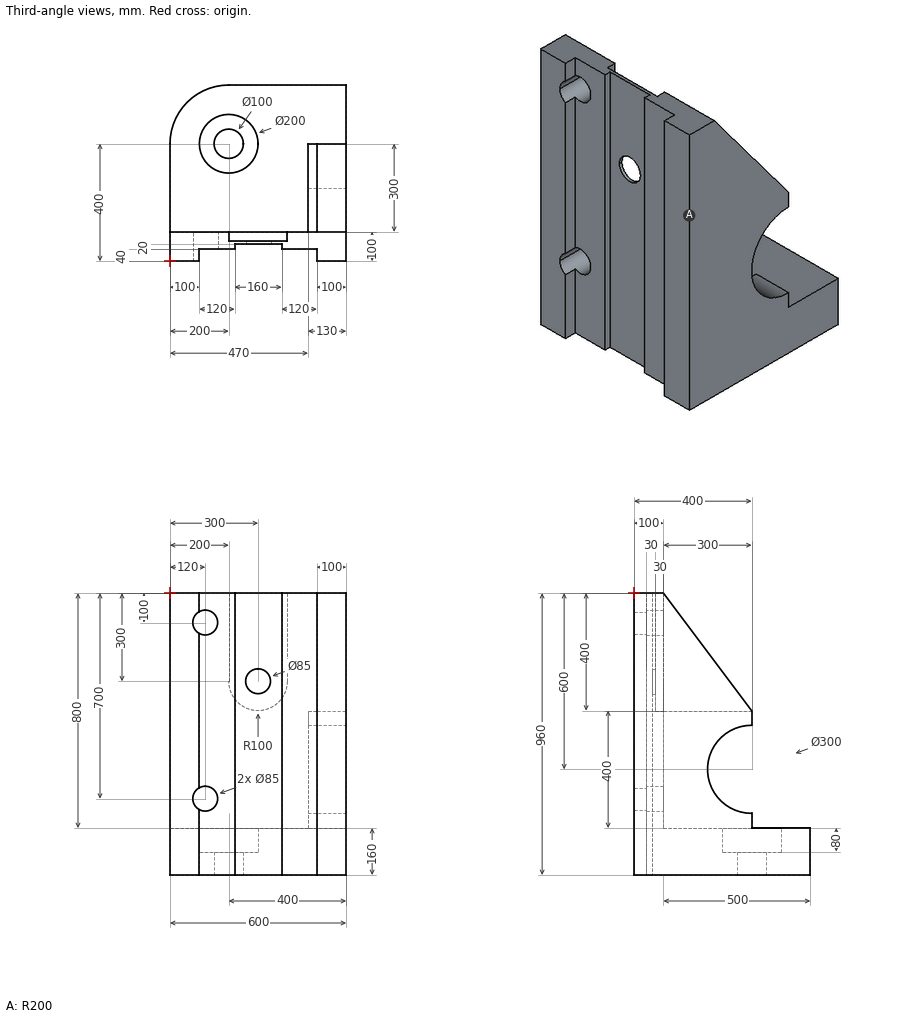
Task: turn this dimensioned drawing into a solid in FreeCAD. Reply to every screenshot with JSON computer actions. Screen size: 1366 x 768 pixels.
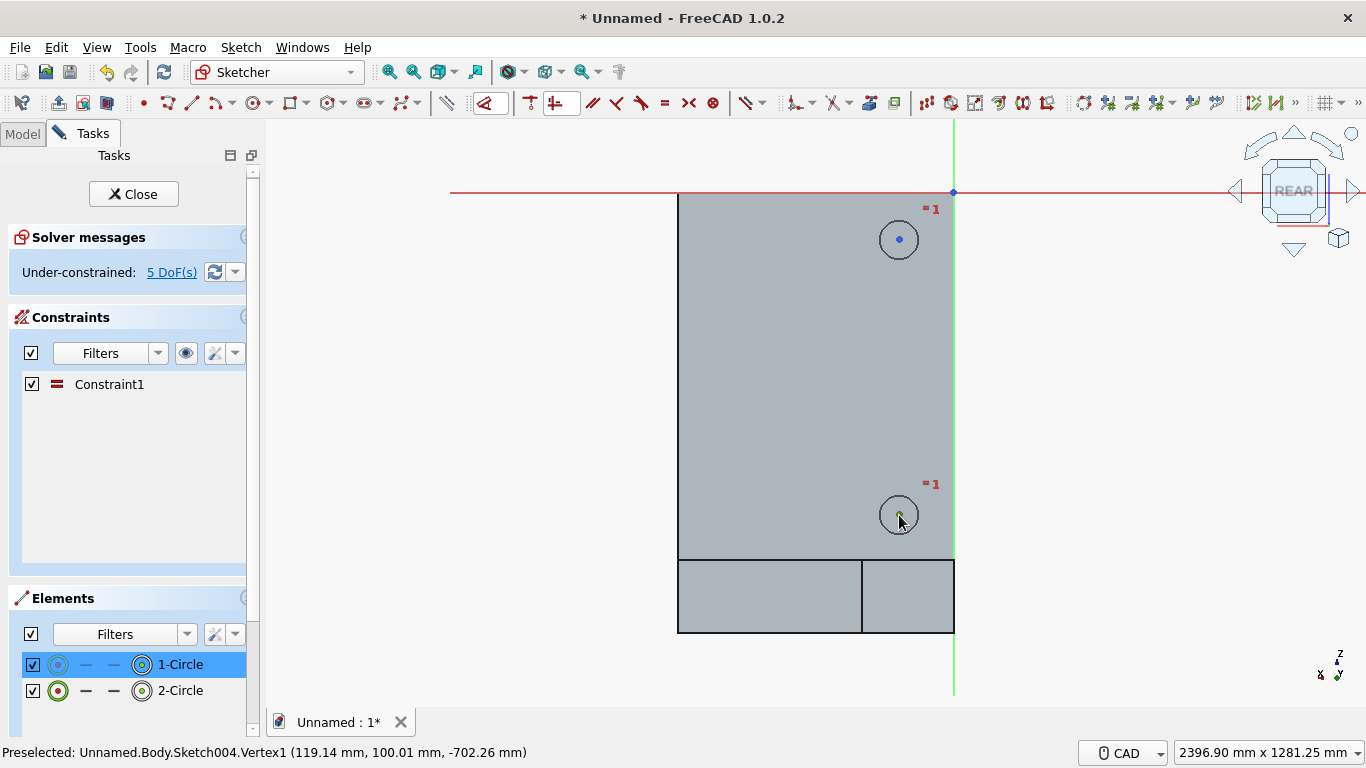
{"action": "left_click", "coordinate": [899, 240]}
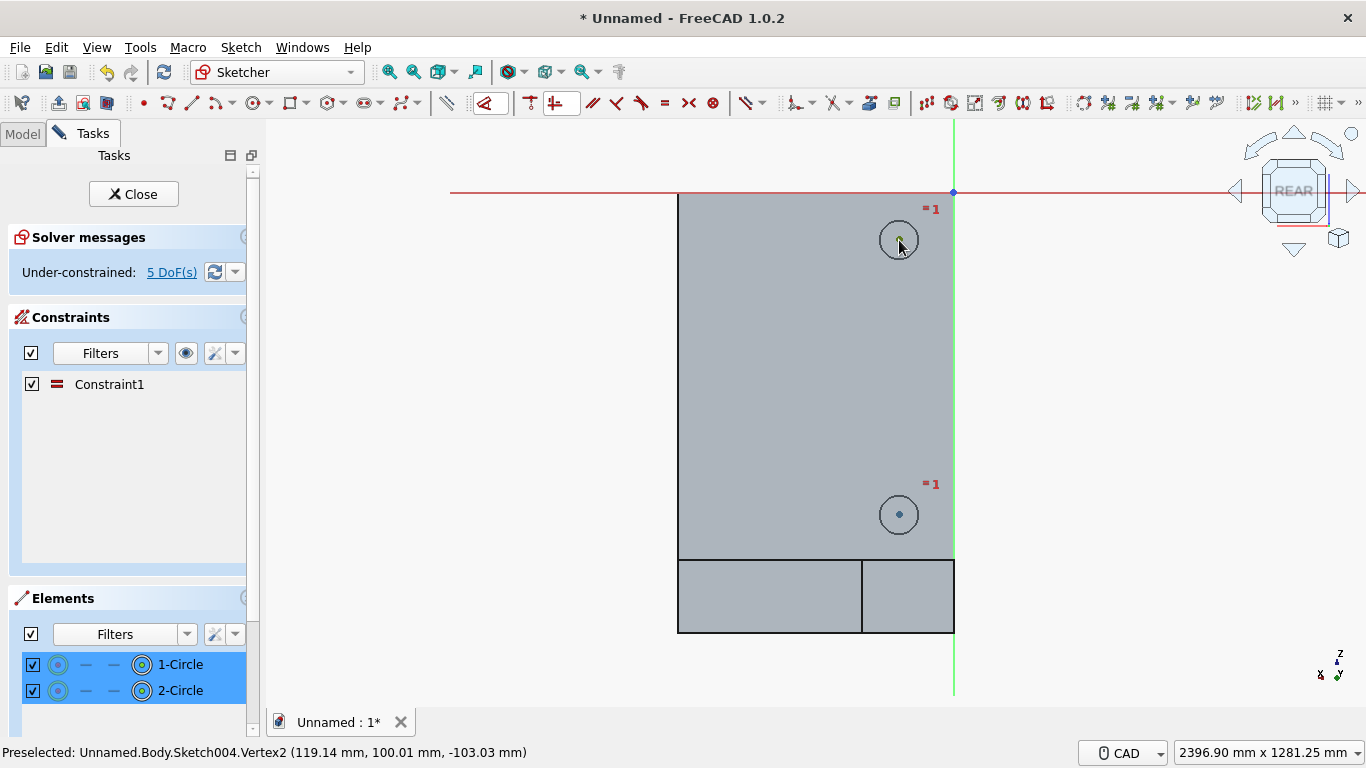
{"action": "key", "text": "v"}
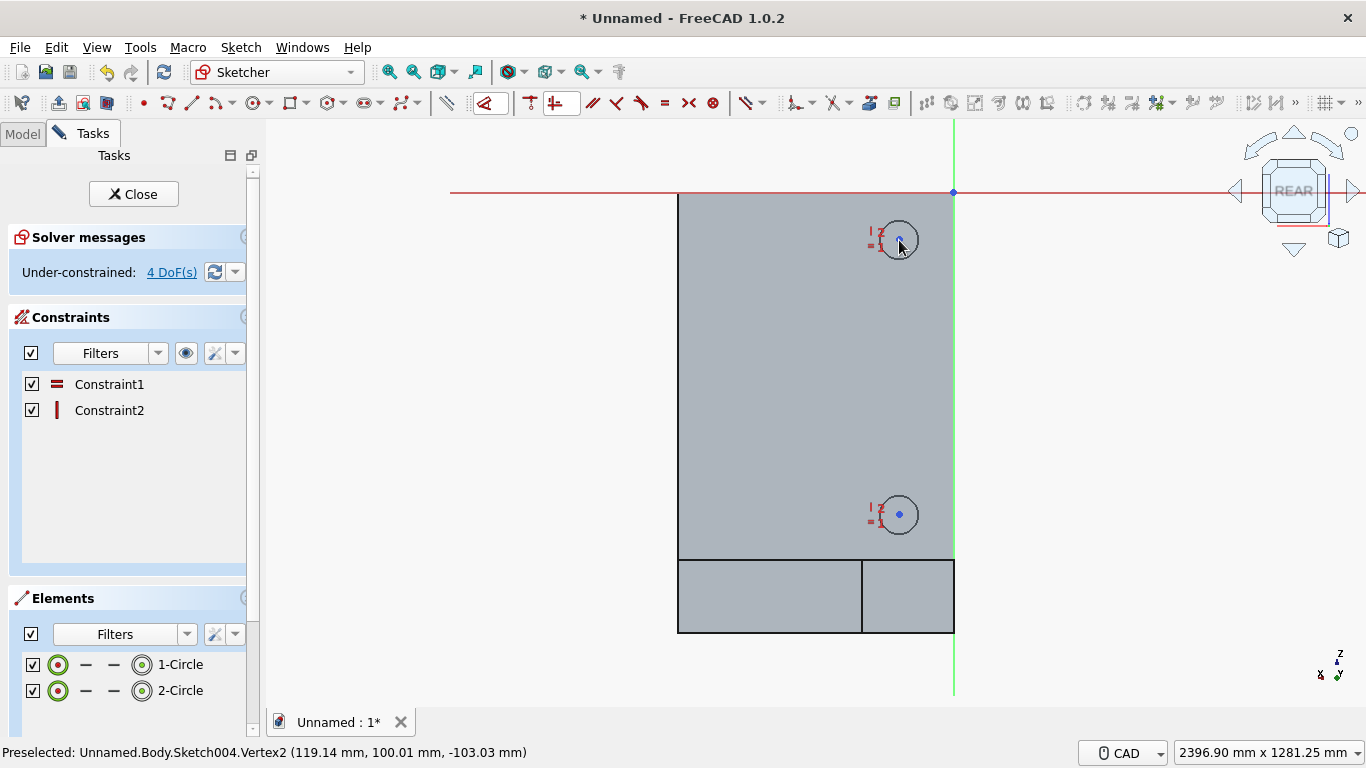
{"action": "left_click", "coordinate": [912, 501]}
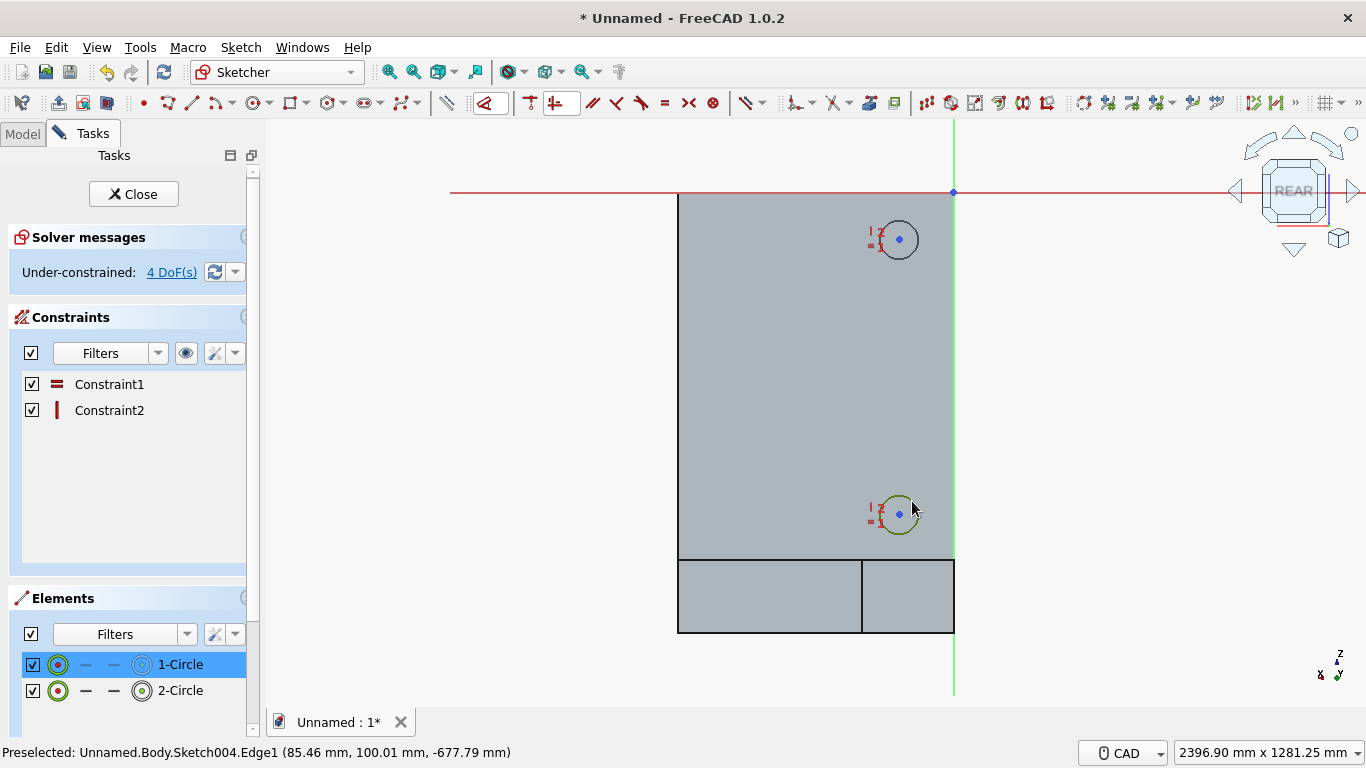
{"action": "key", "text": "k o"}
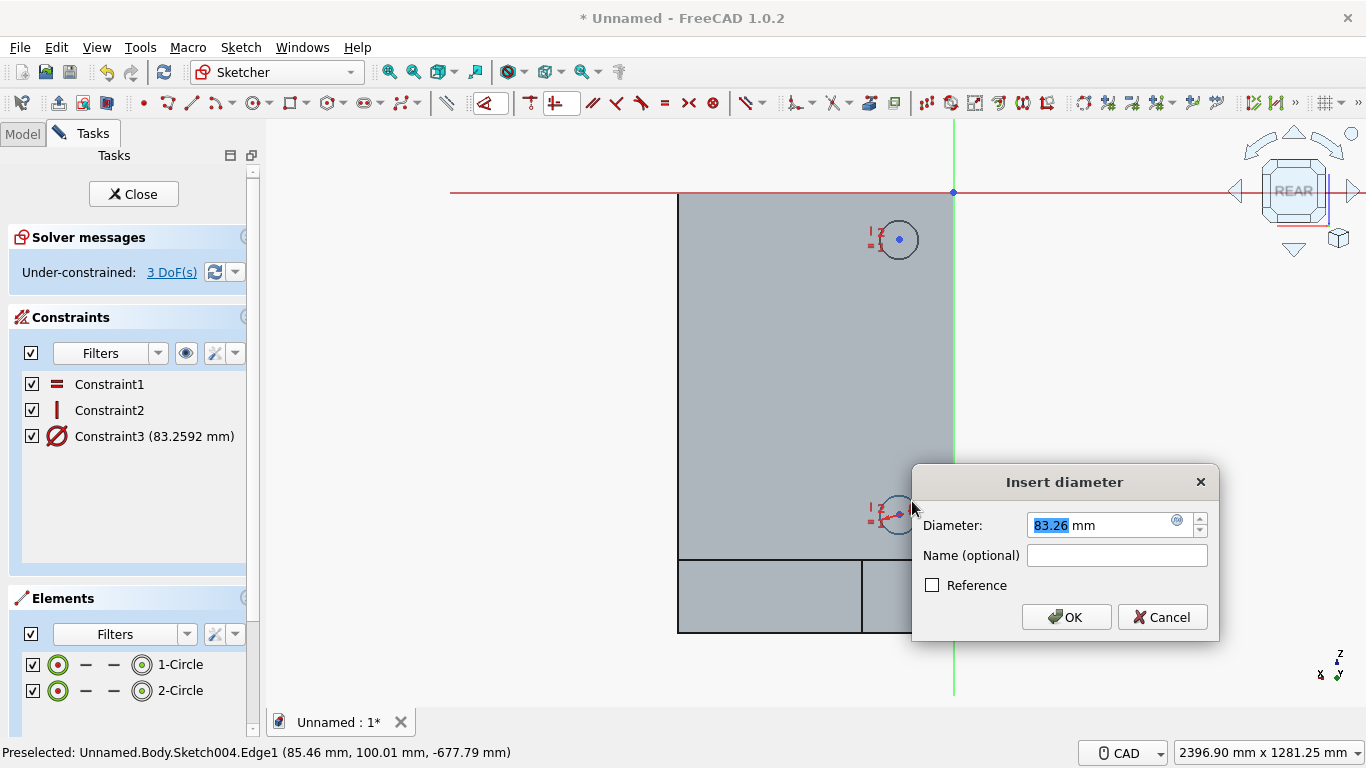
{"action": "type", "text": "85"}
{"action": "key", "text": "Return"}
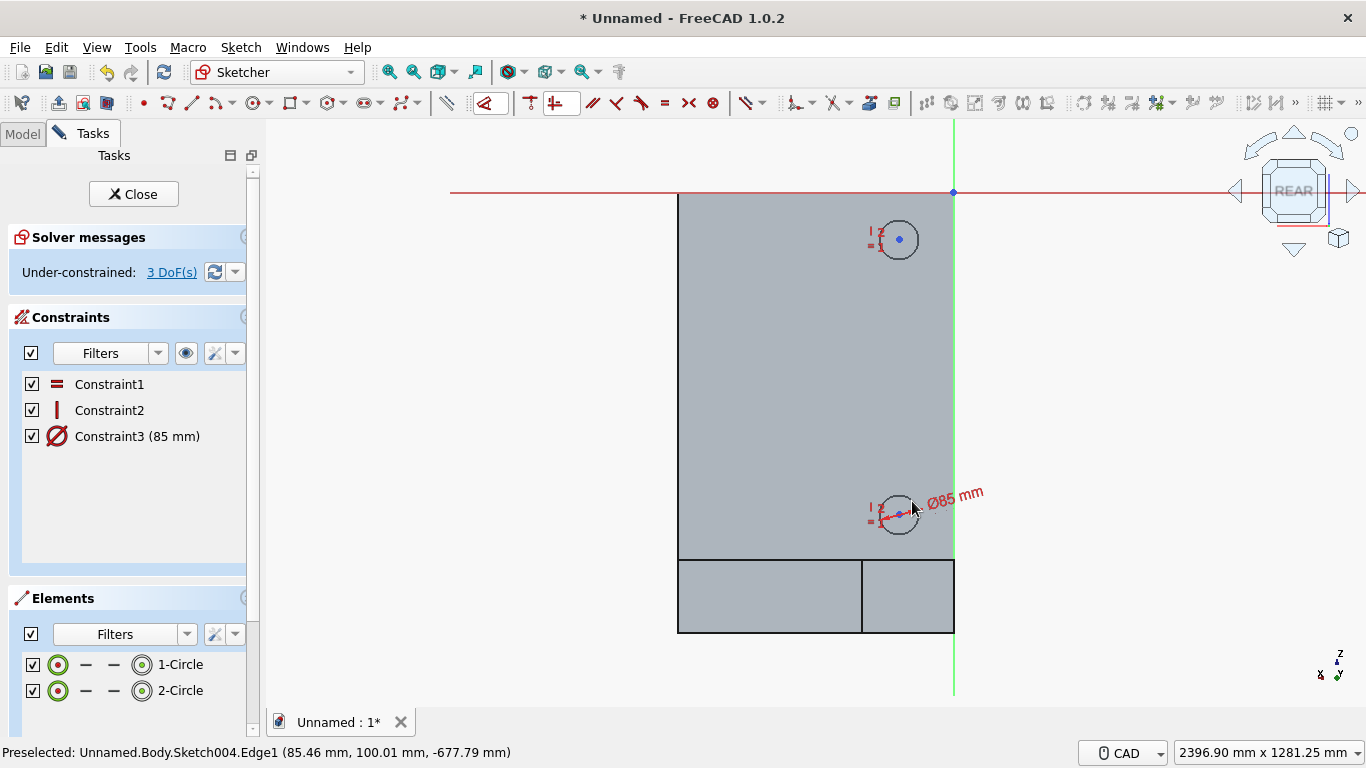
{"action": "left_click", "coordinate": [899, 515]}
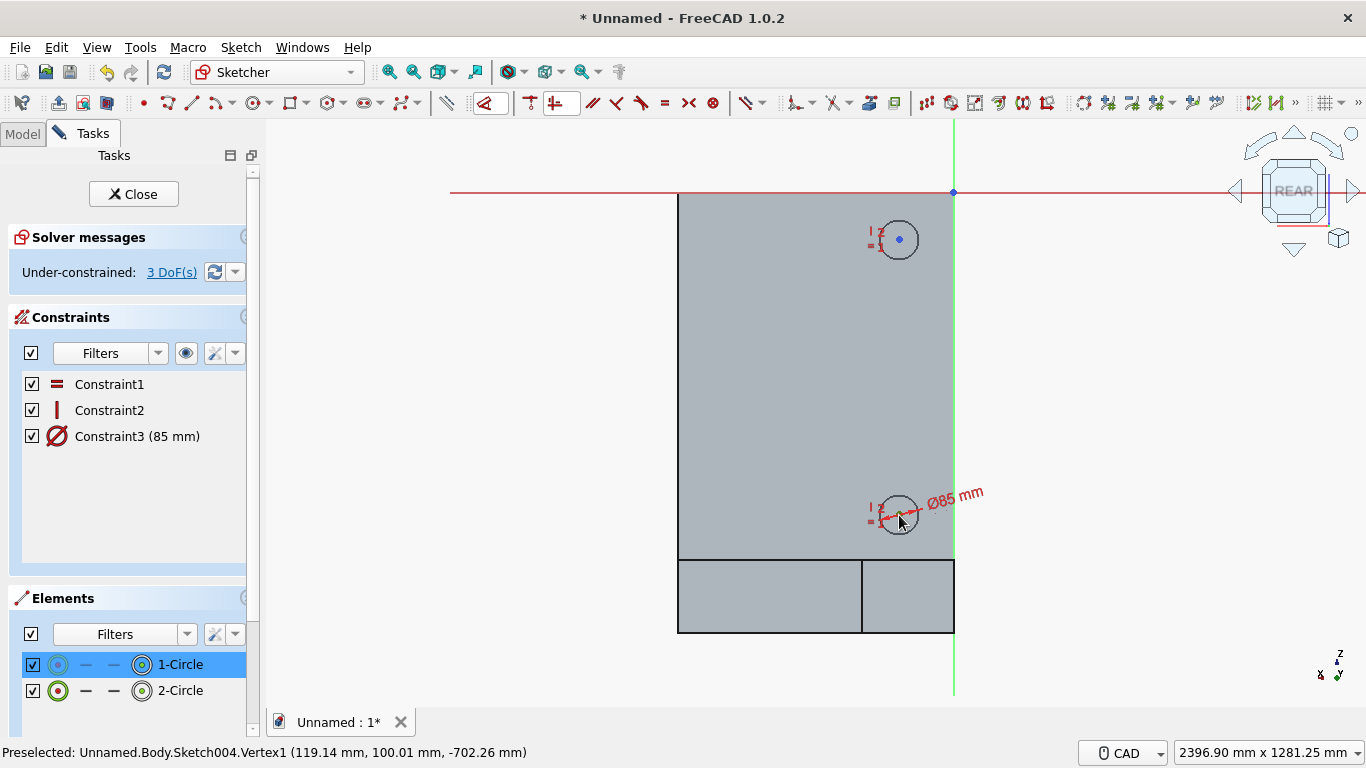
{"action": "left_click", "coordinate": [502, 104]}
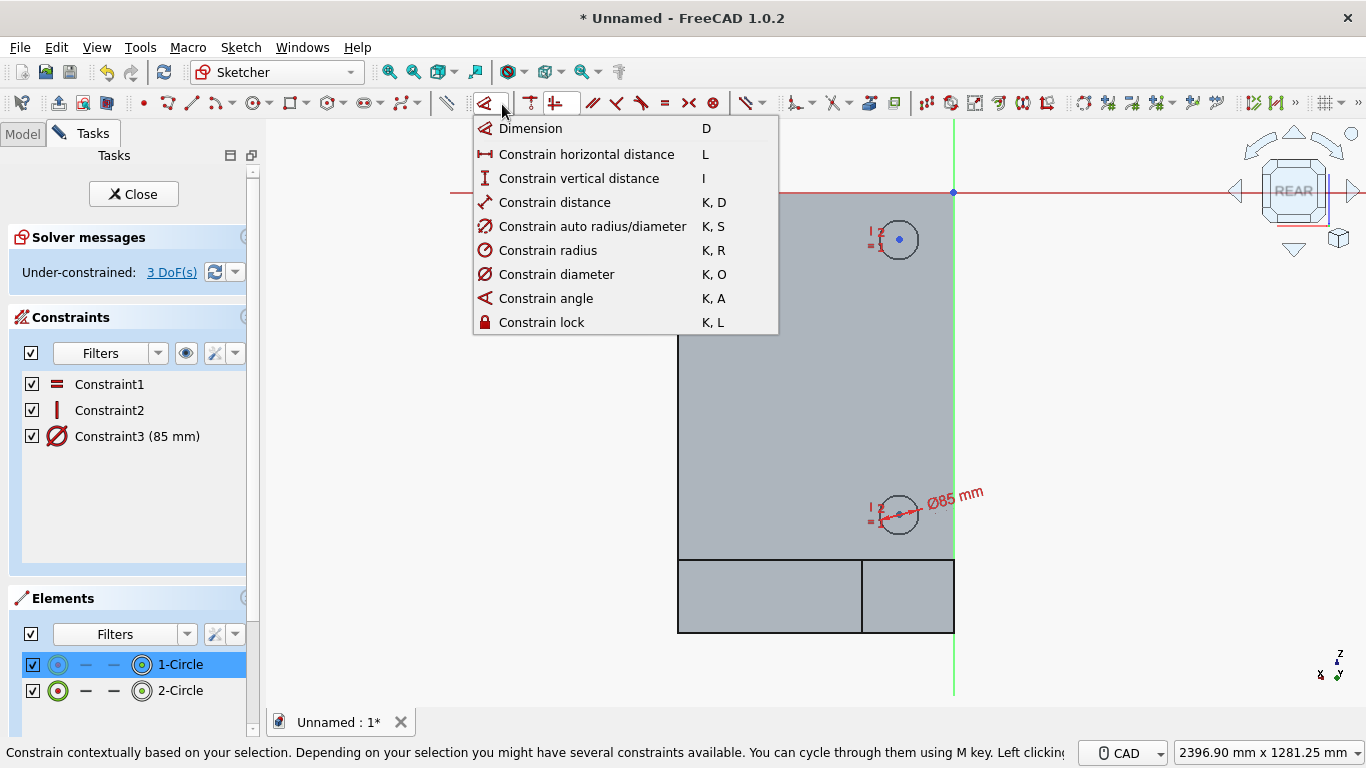
{"action": "left_click", "coordinate": [626, 154]}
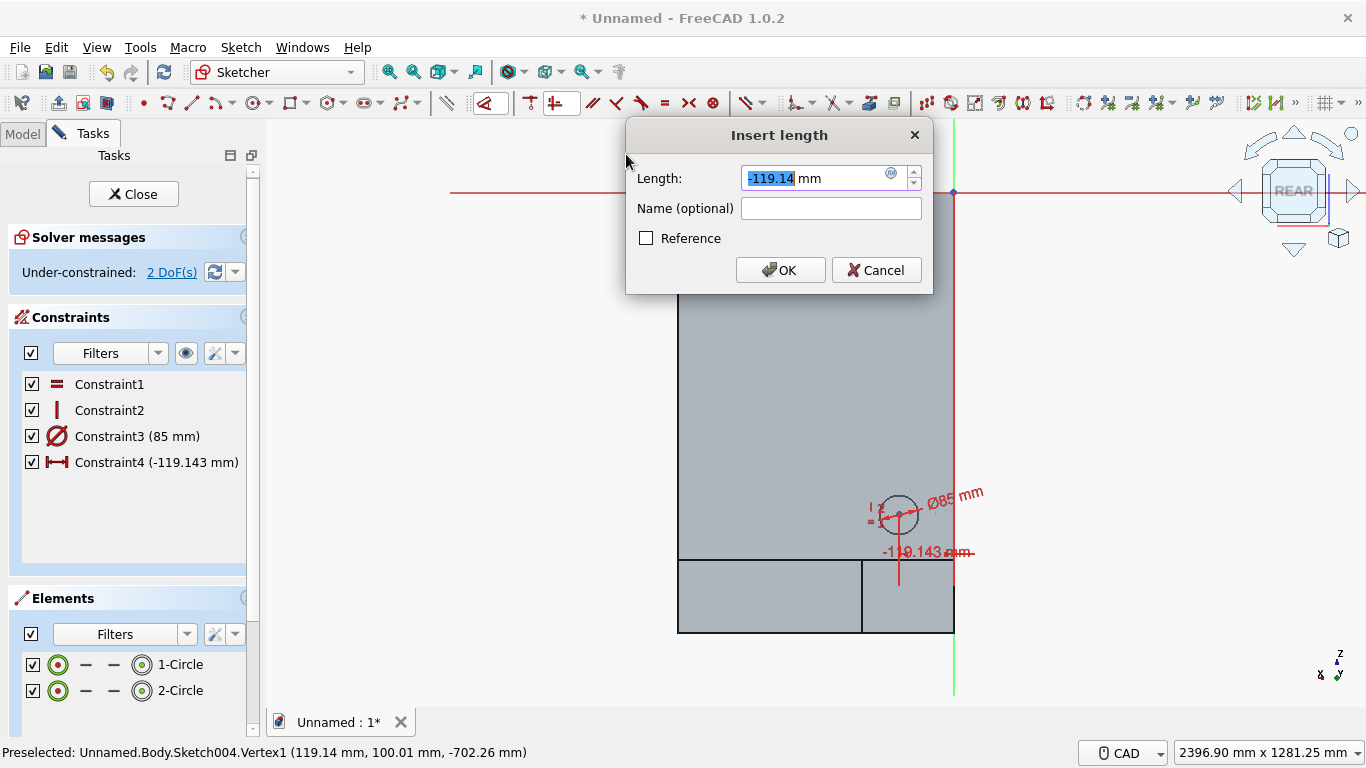
{"action": "type", "text": "-120"}
{"action": "key", "text": "Return"}